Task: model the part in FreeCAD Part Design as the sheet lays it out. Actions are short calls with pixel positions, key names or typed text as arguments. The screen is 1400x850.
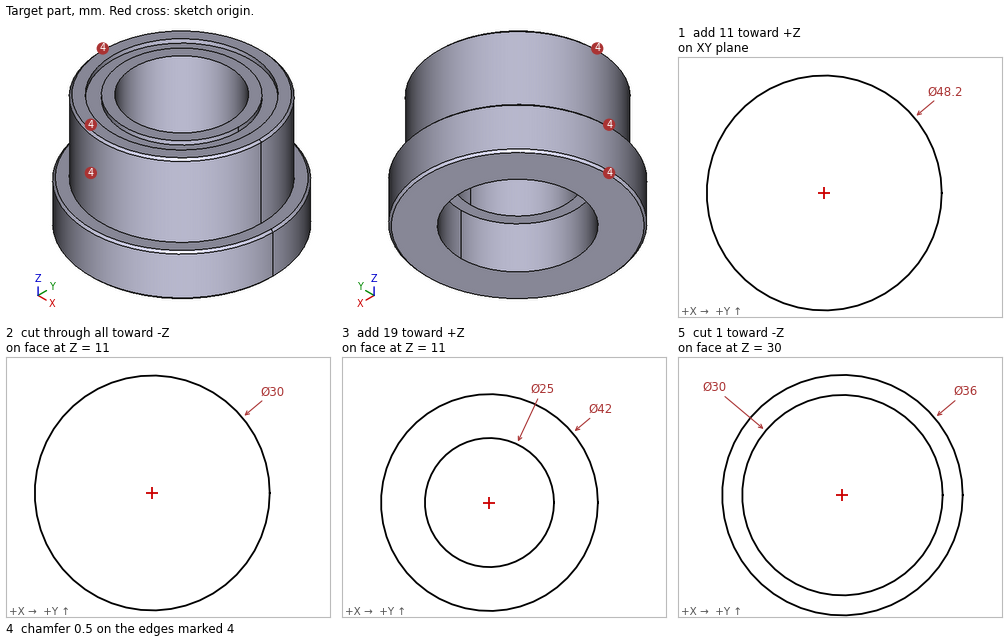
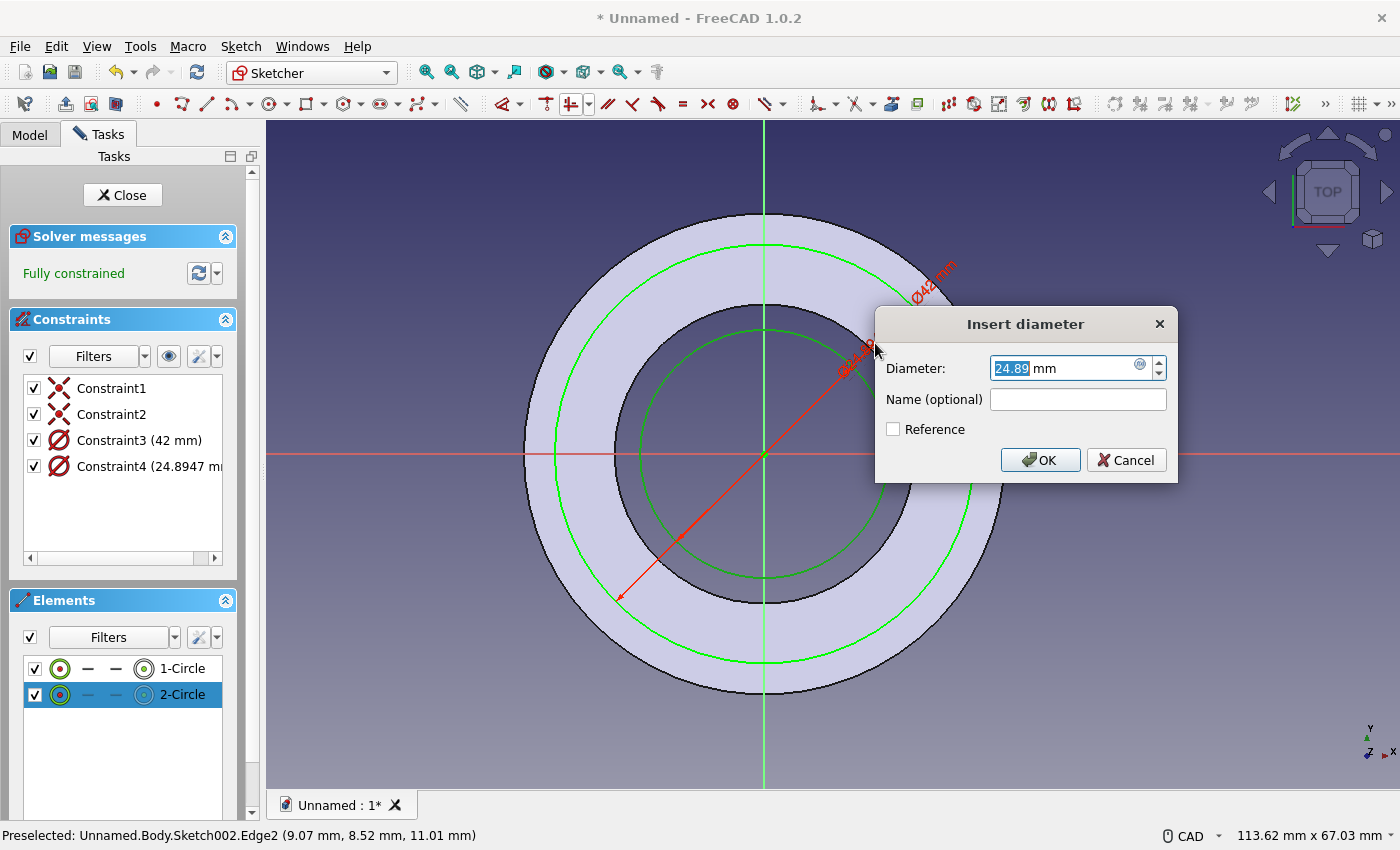
text(25)
key(Return)
key(Escape)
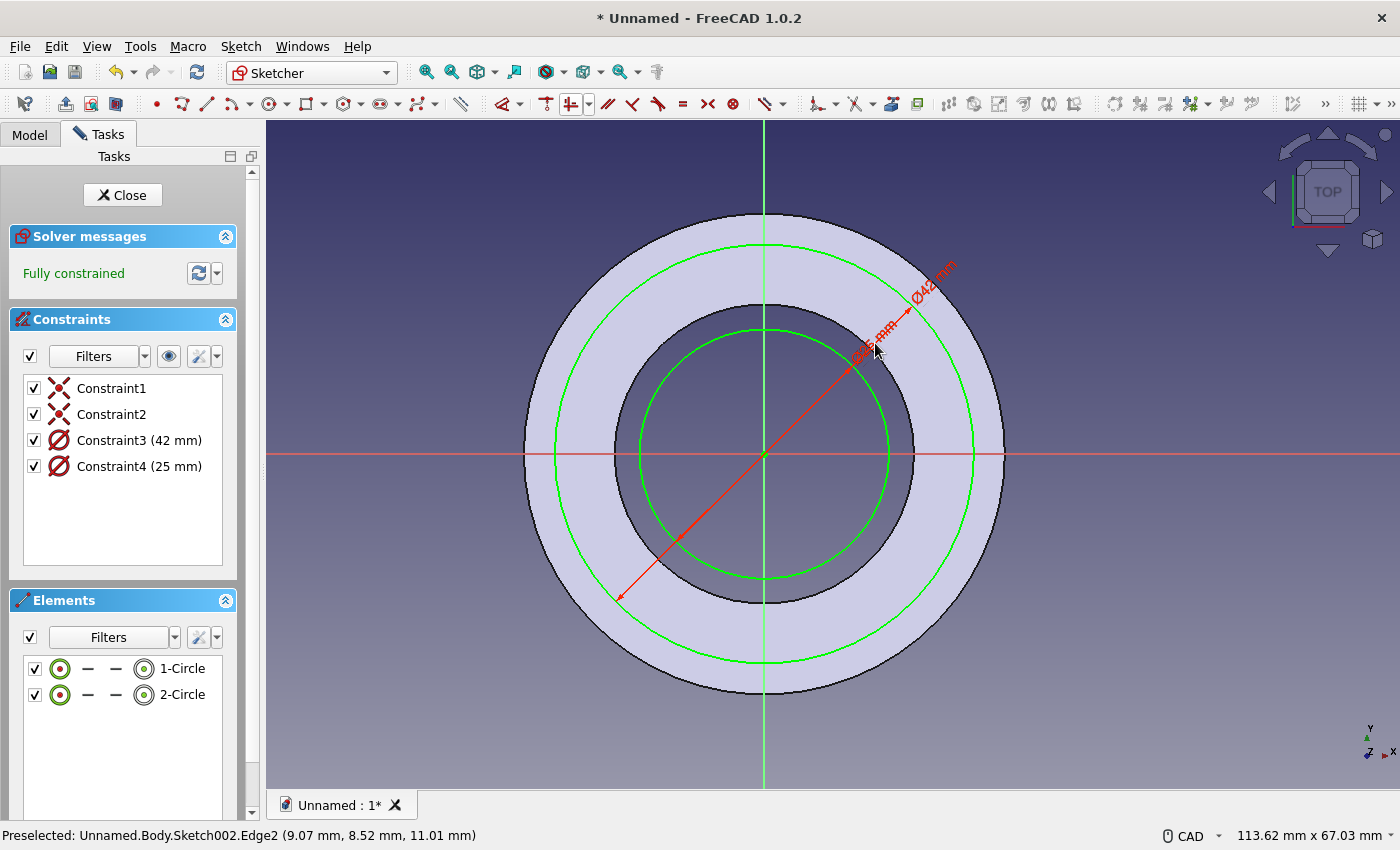
click(123, 195)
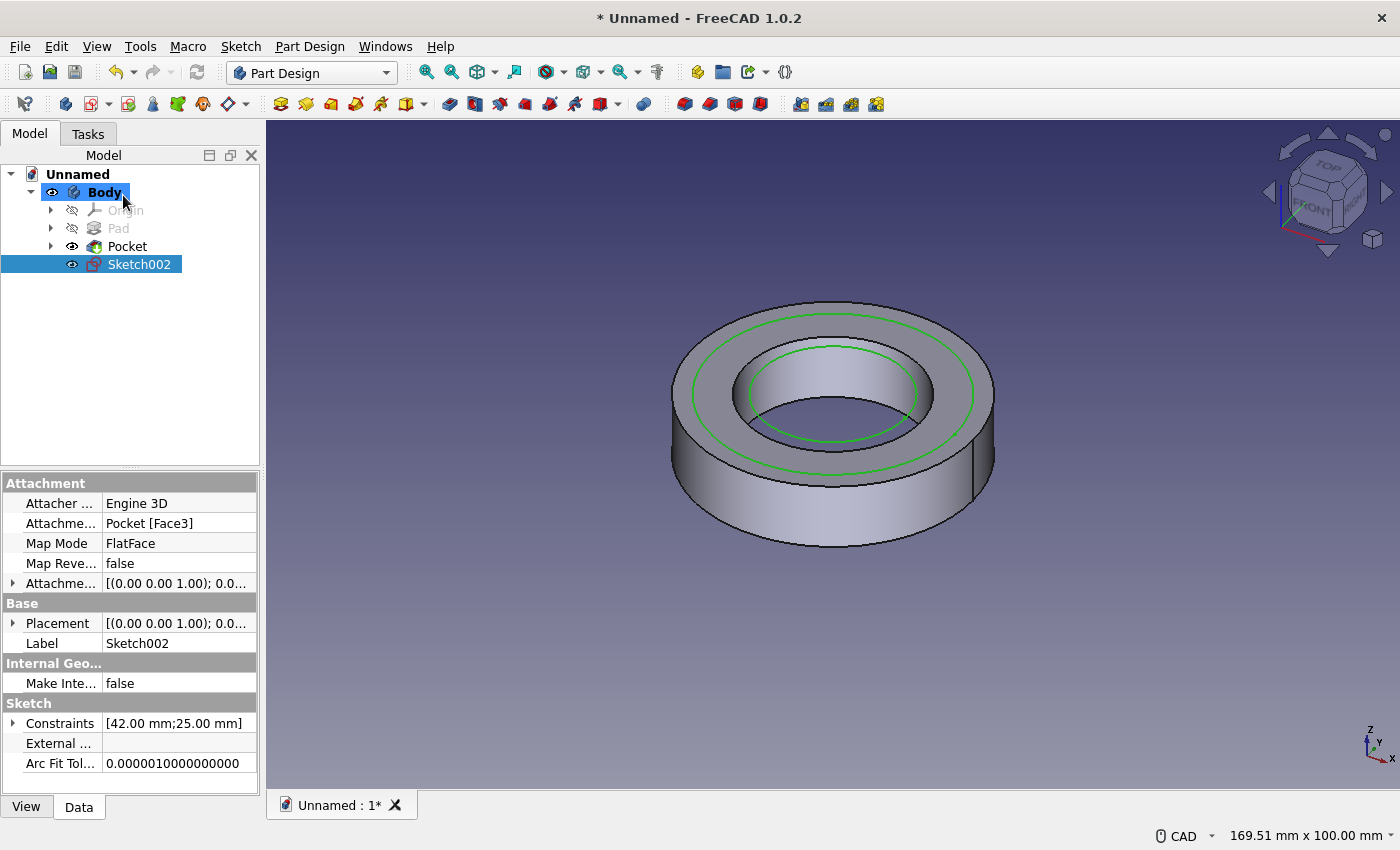
click(281, 104)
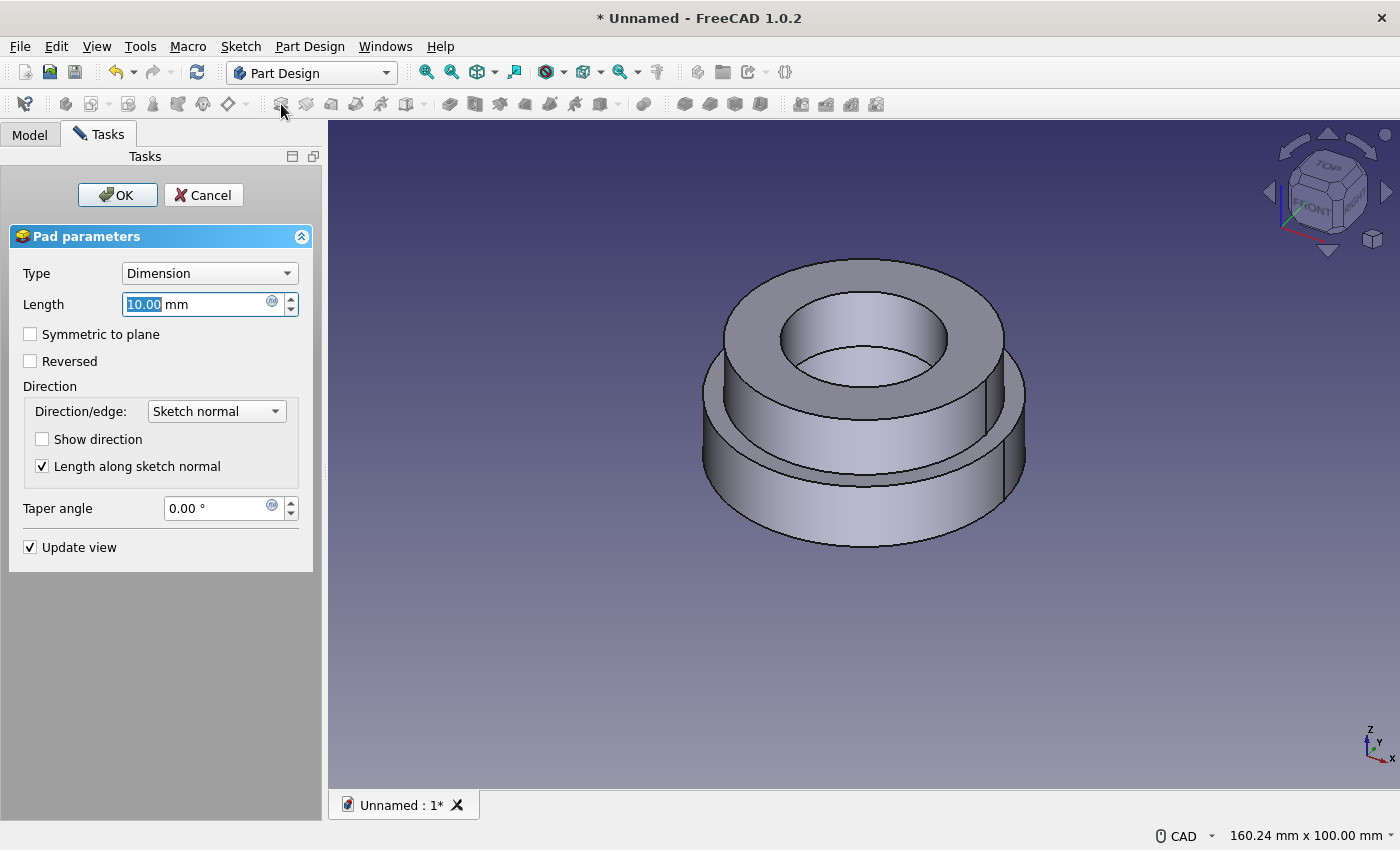
text(19)
key(Tab)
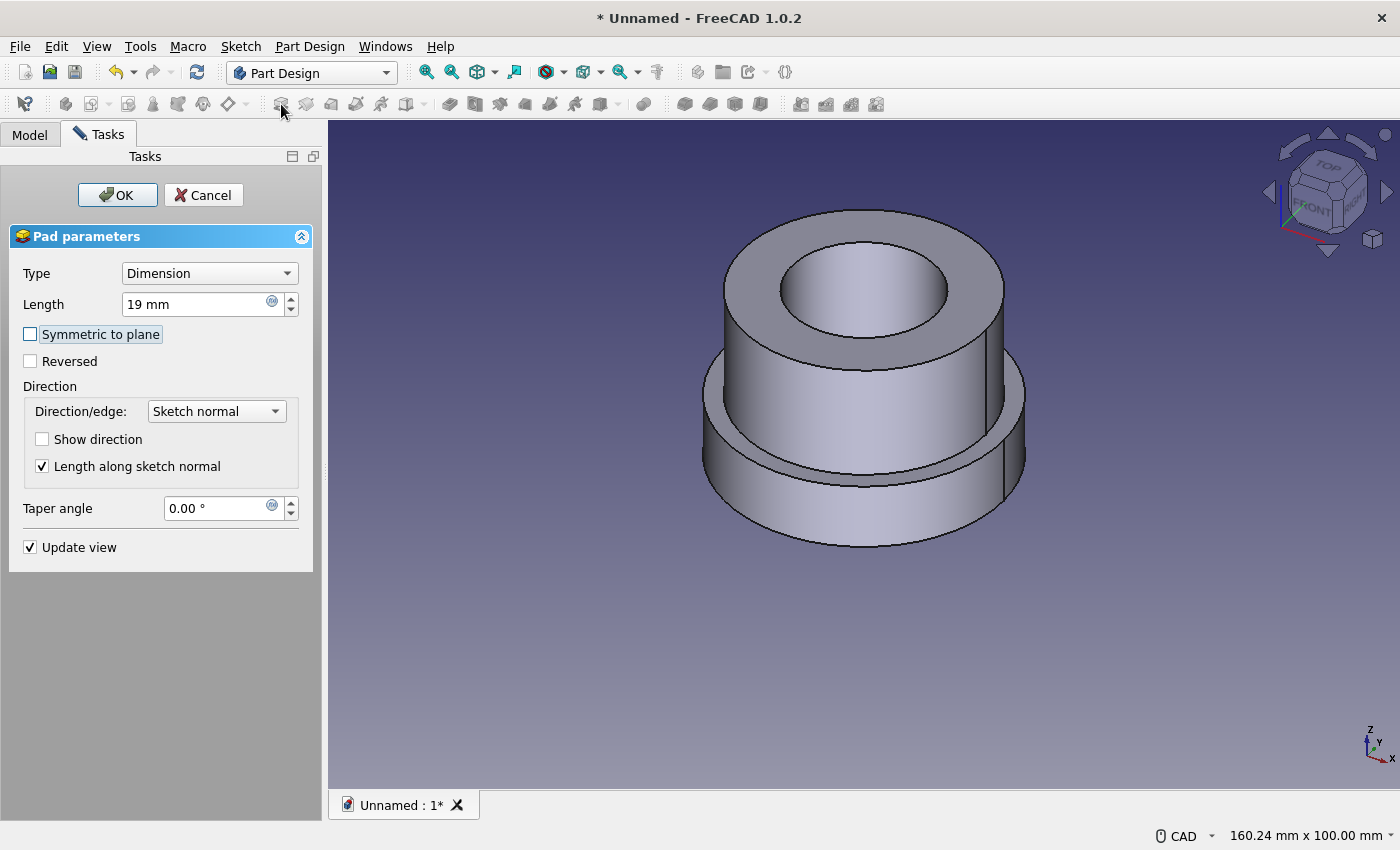
click(118, 195)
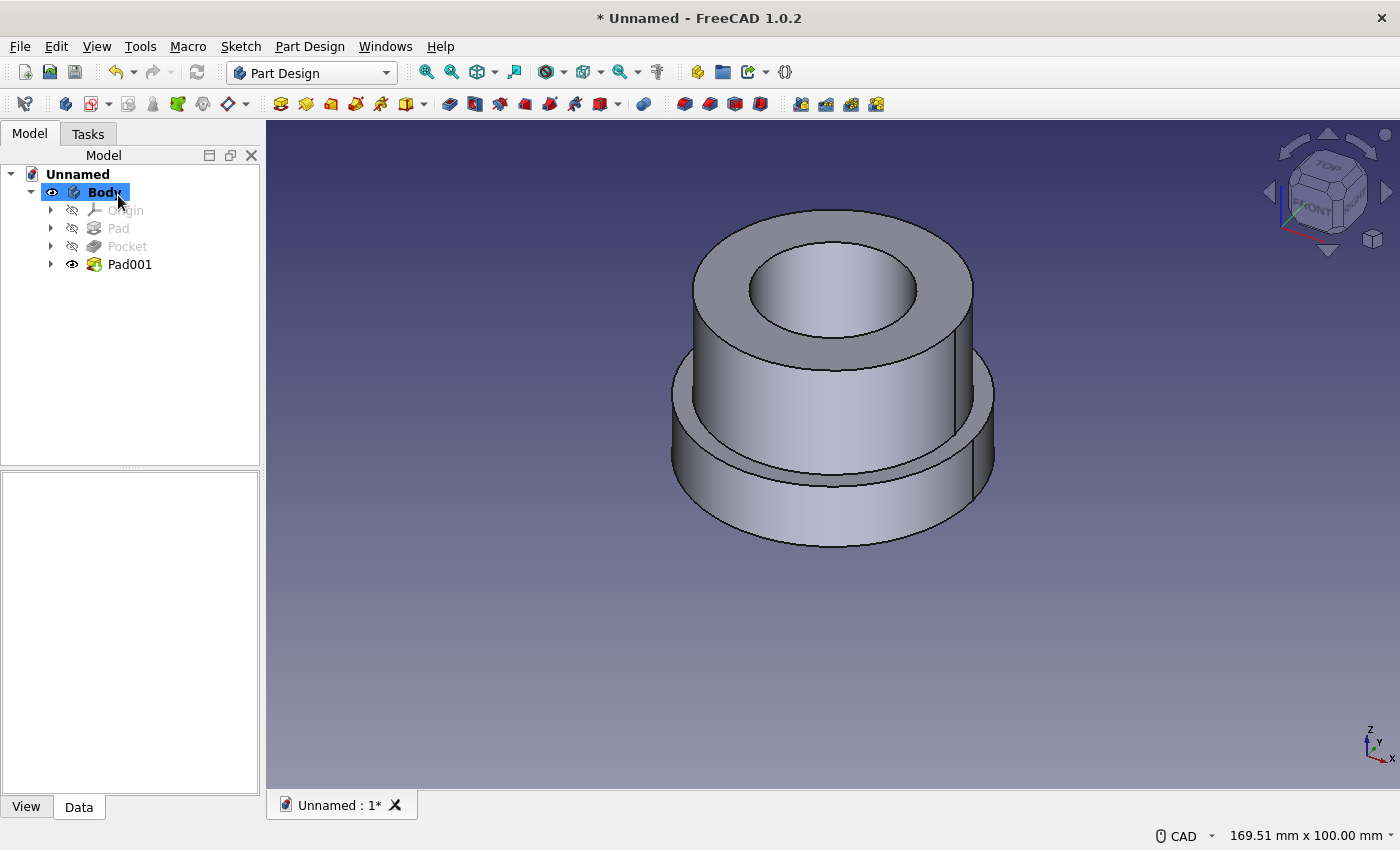
click(693, 298)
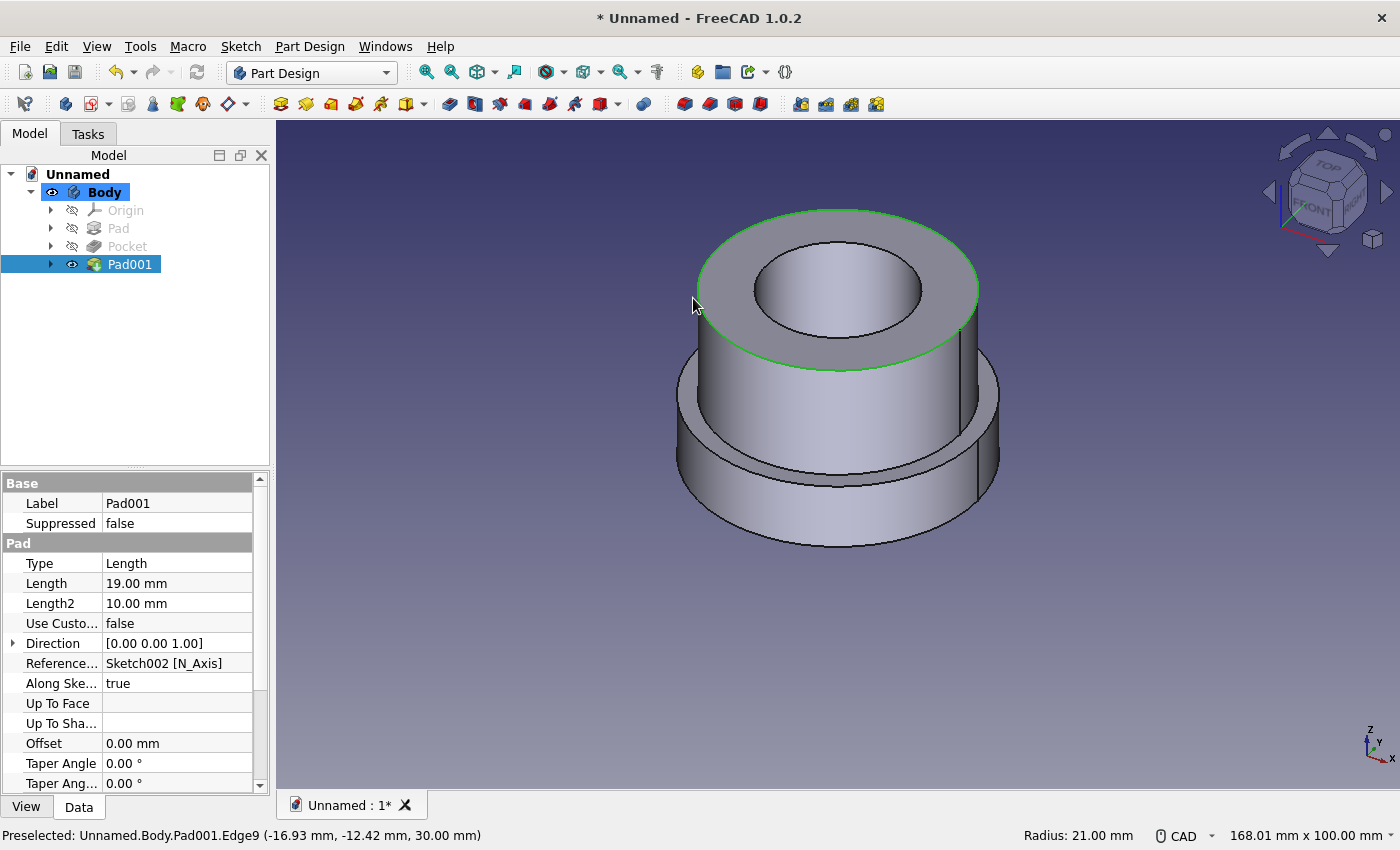
click(678, 403, ctrl)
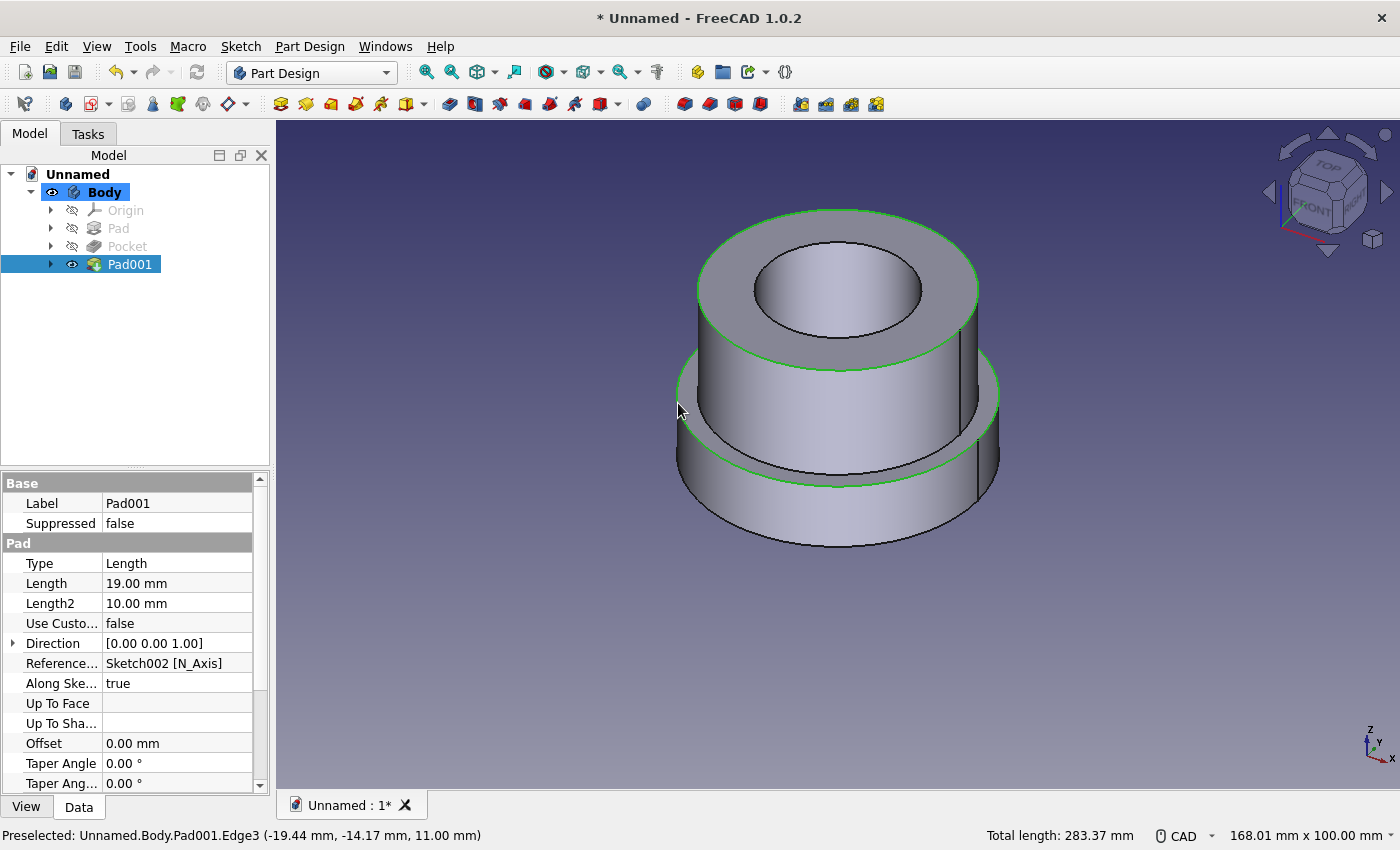
key(0)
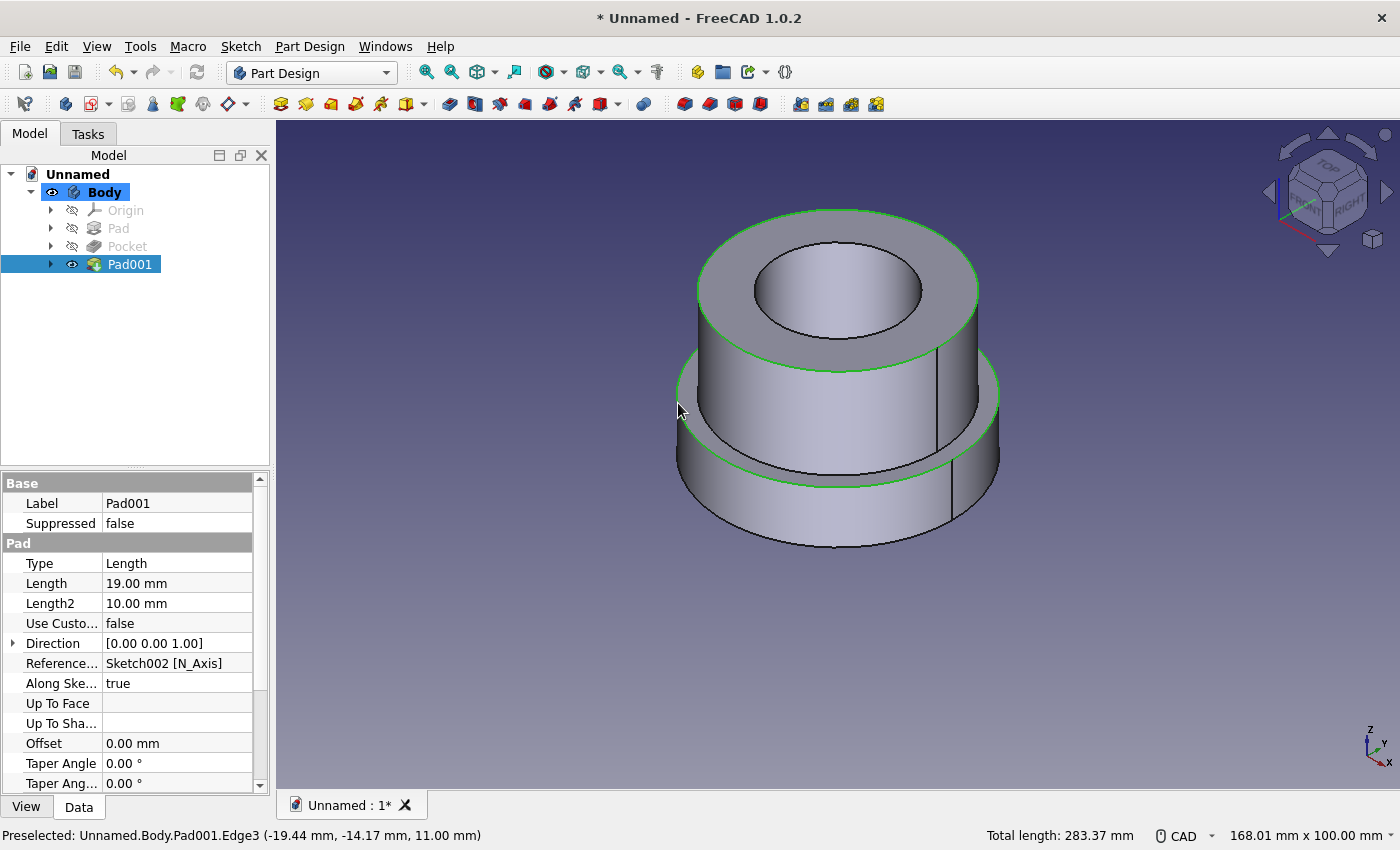
click(694, 496, ctrl)